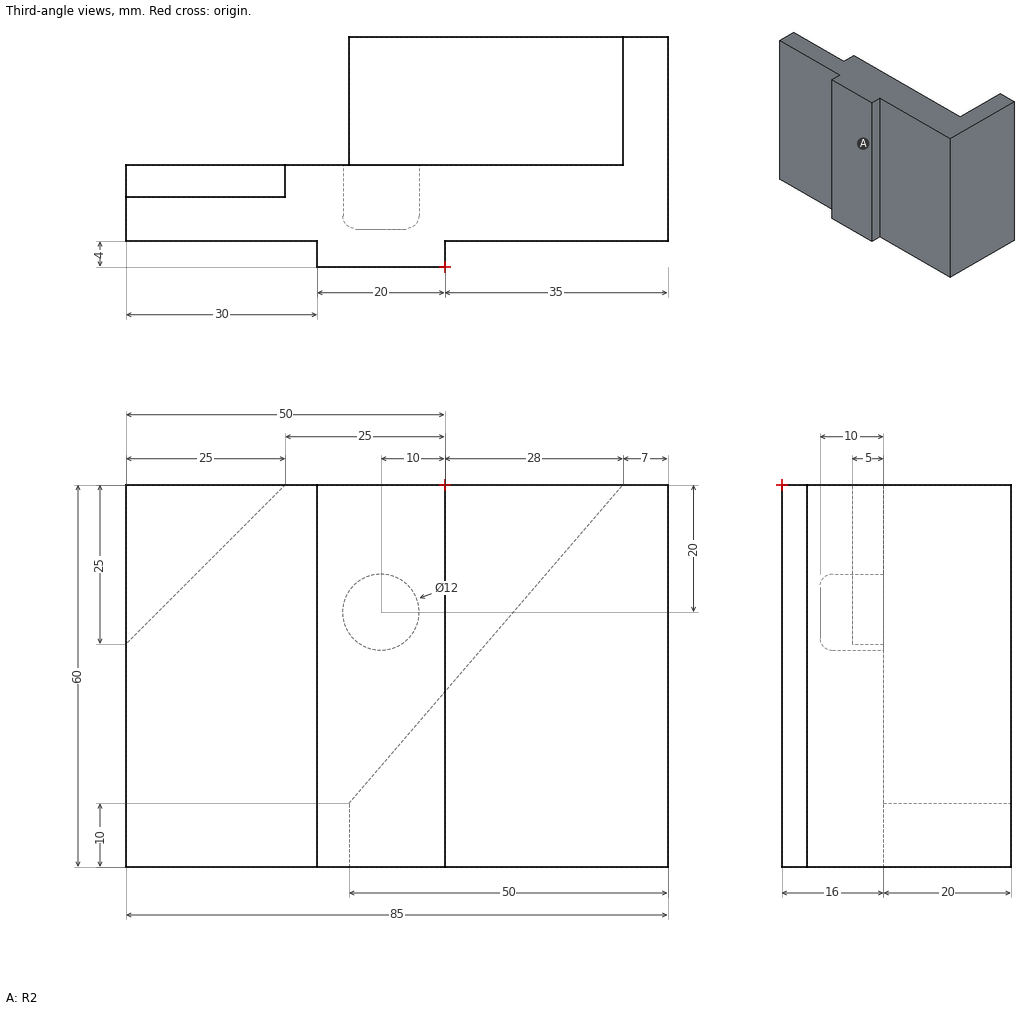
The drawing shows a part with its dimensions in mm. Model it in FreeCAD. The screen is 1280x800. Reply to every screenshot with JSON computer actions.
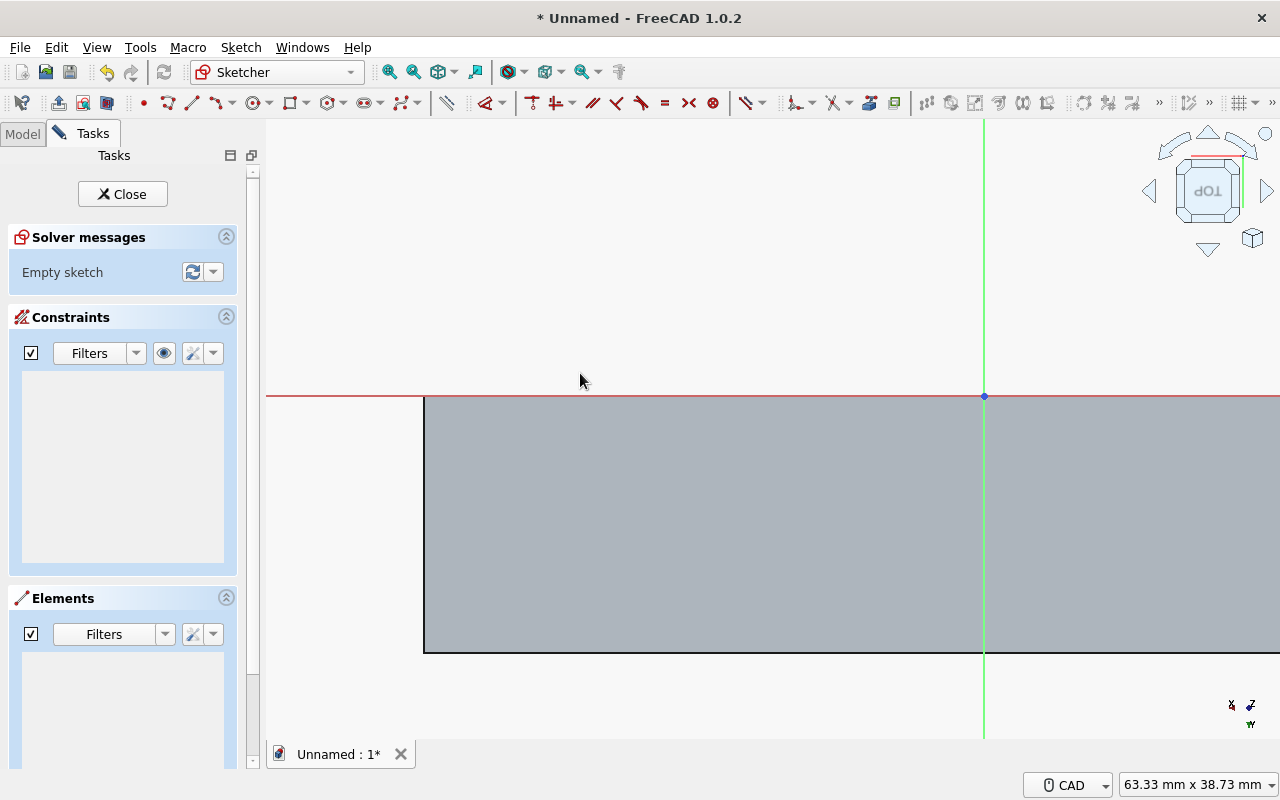
{"action": "left_click", "coordinate": [290, 104]}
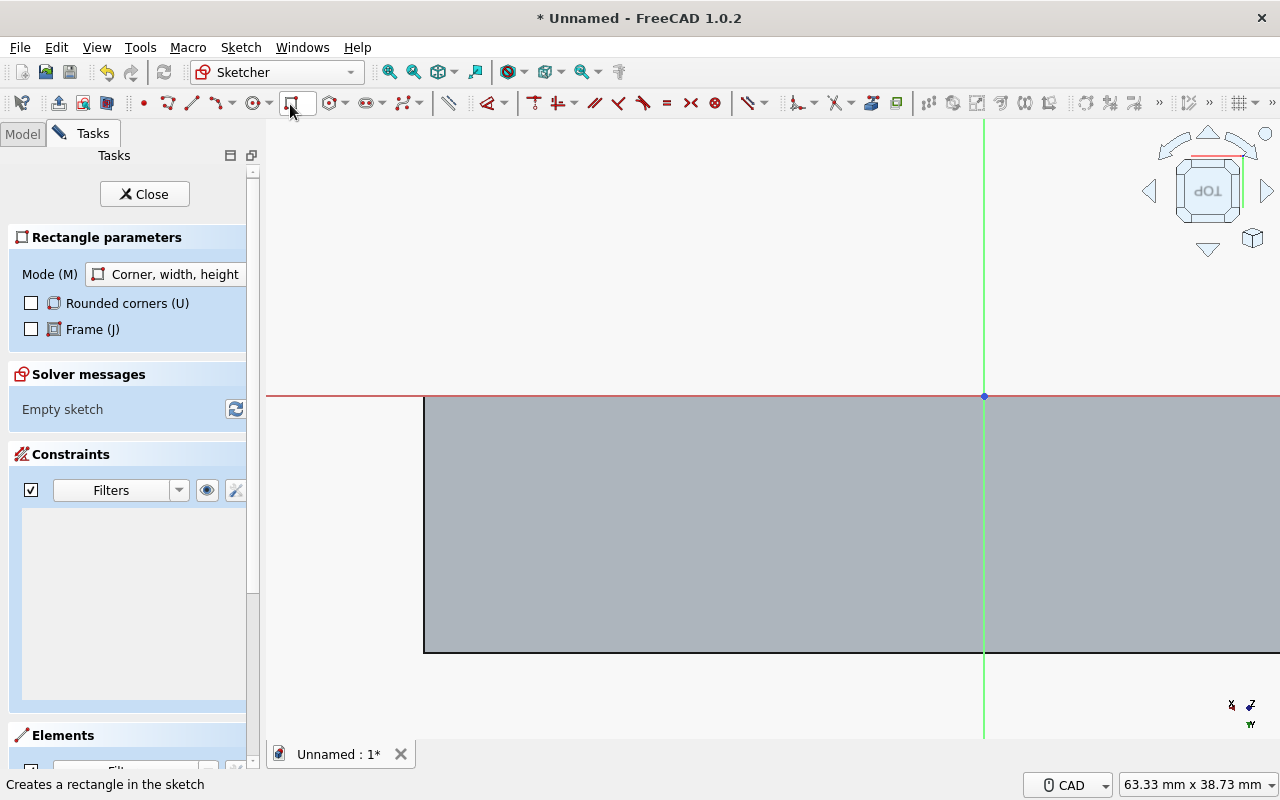
{"action": "left_click", "coordinate": [984, 396]}
{"action": "left_click", "coordinate": [424, 460]}
{"action": "key", "text": "Escape"}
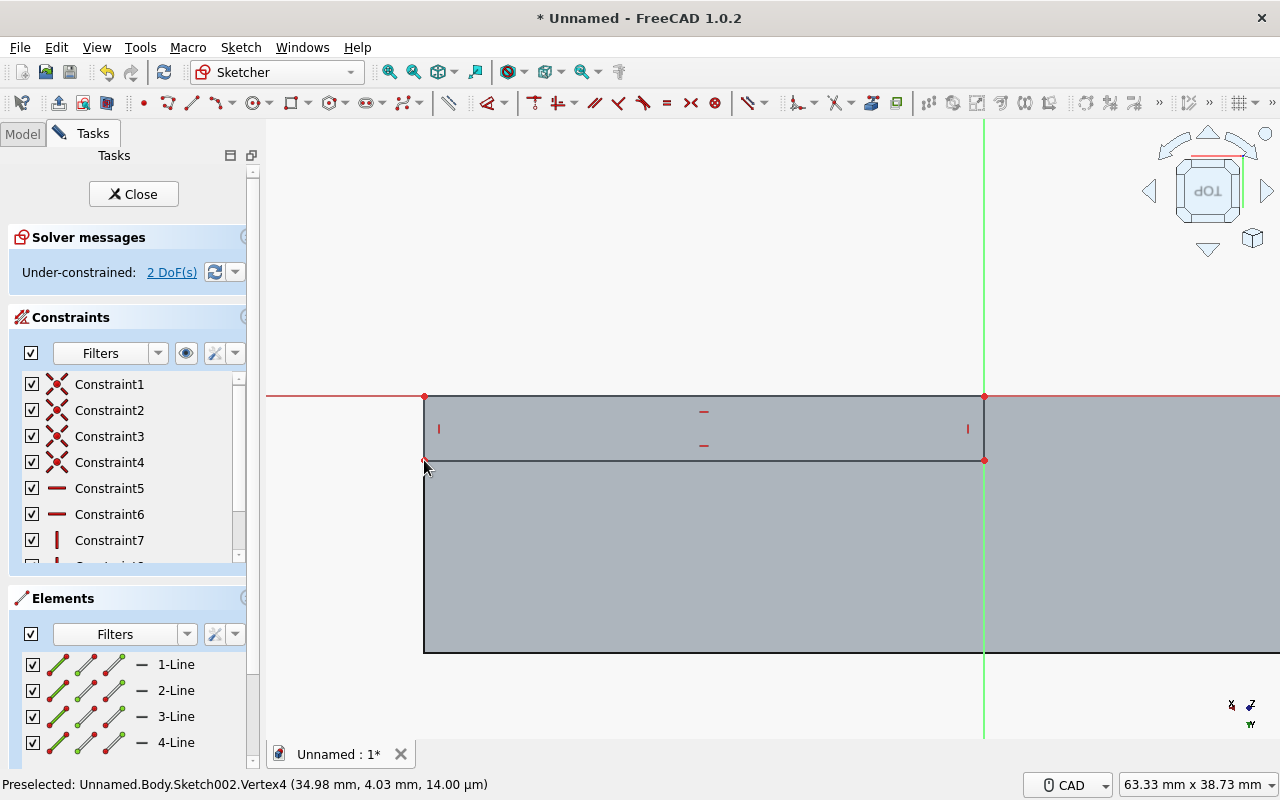
{"action": "left_click", "coordinate": [488, 104]}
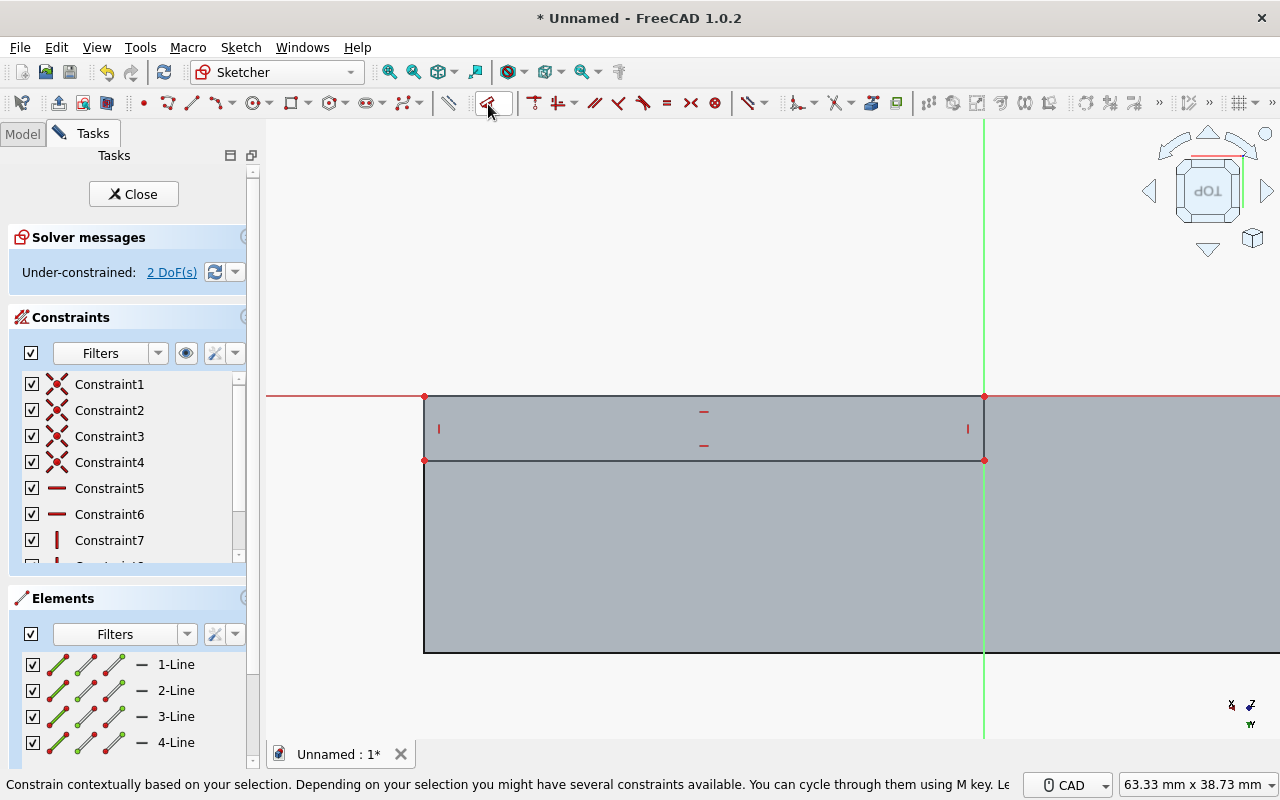
{"action": "left_click", "coordinate": [424, 416]}
{"action": "left_click", "coordinate": [390, 429]}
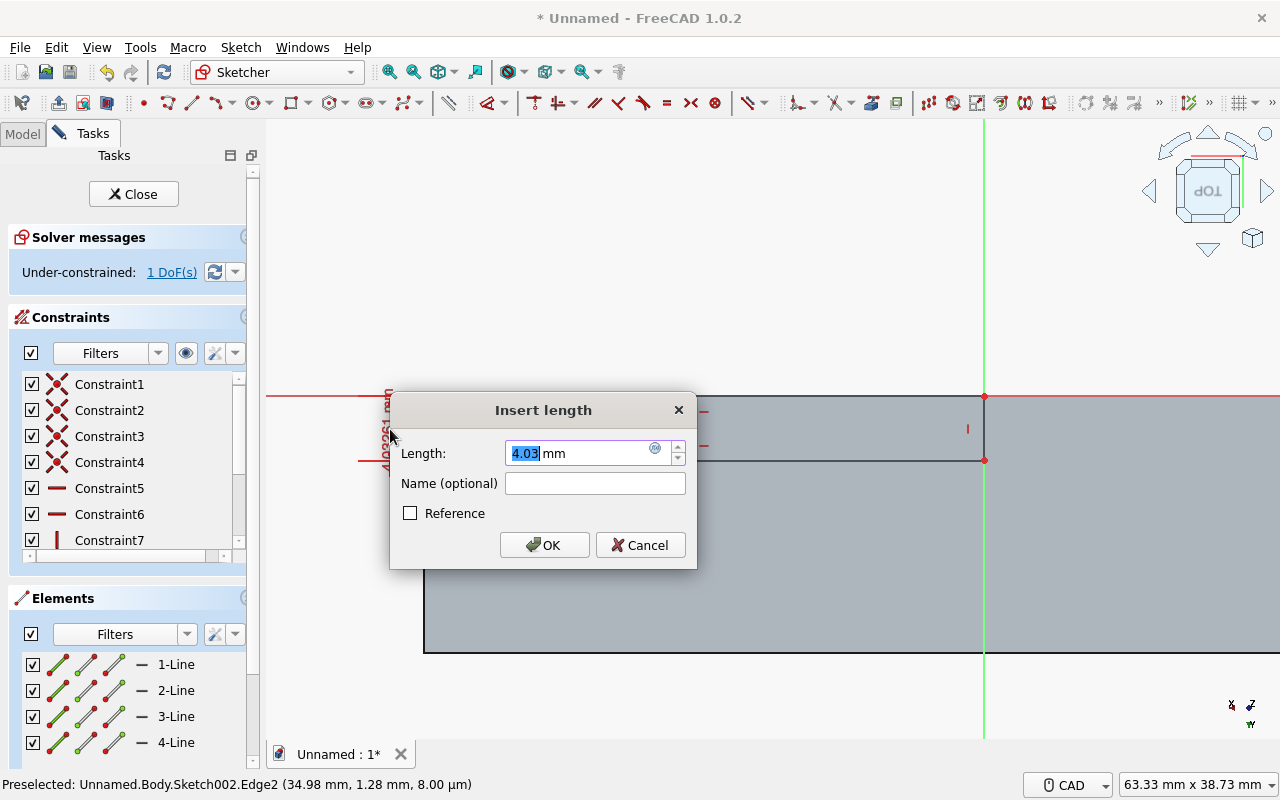
{"action": "type", "text": "4"}
{"action": "key", "text": "Return"}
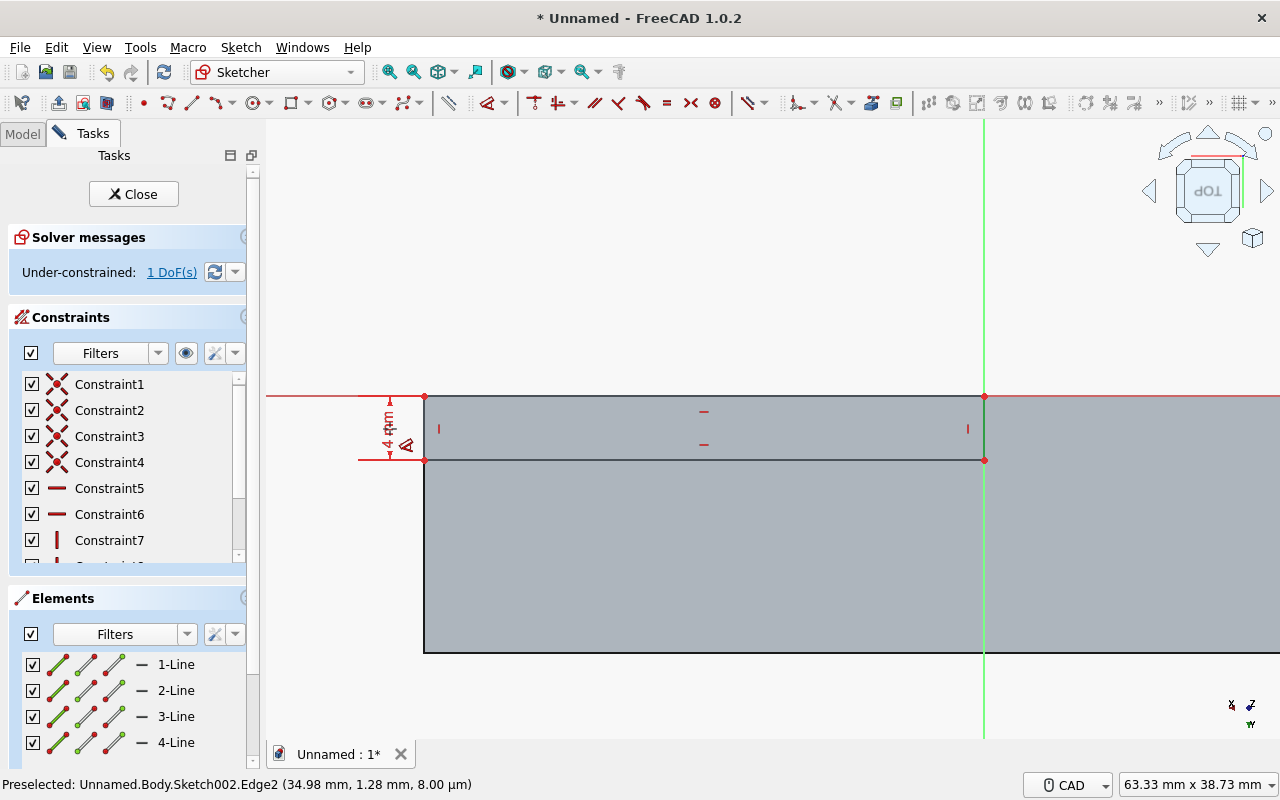
{"action": "left_click", "coordinate": [816, 396]}
{"action": "left_click", "coordinate": [704, 362]}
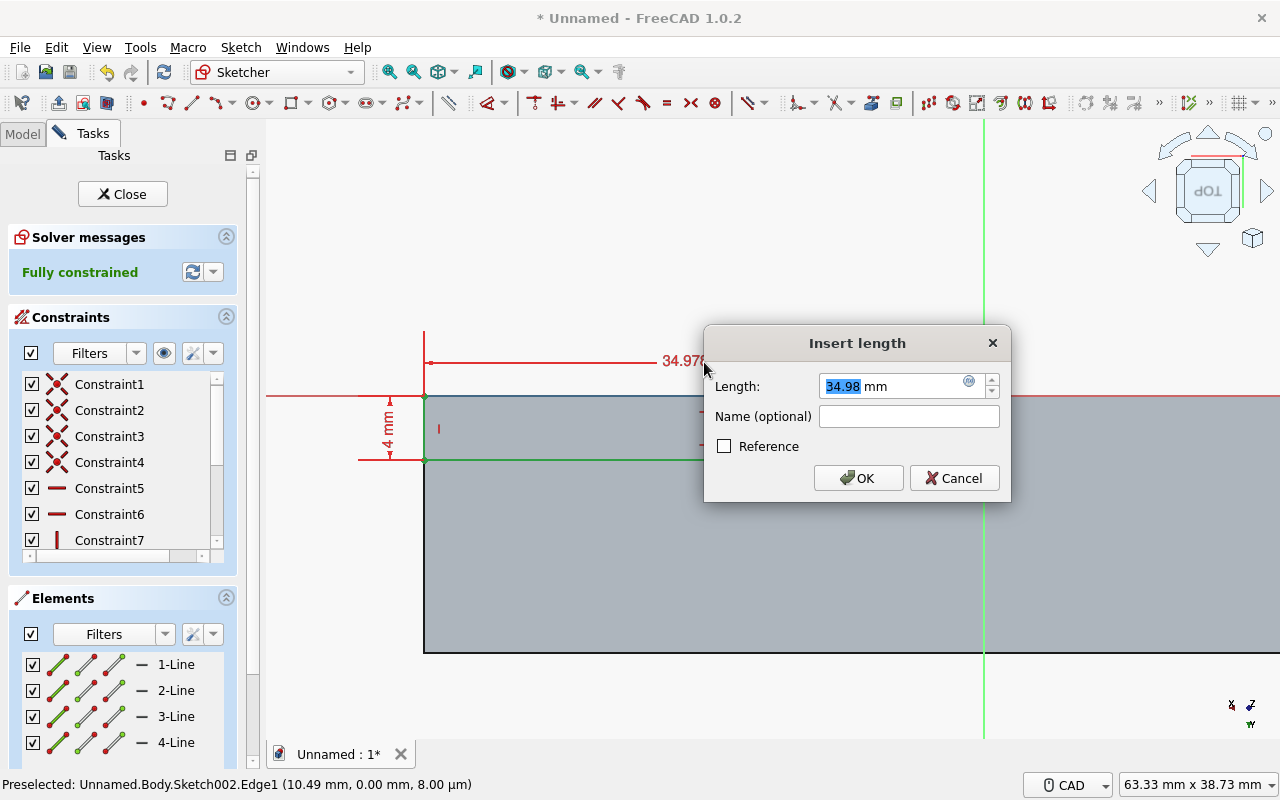
{"action": "type", "text": "35"}
{"action": "key", "text": "Return"}
{"action": "key", "text": "Escape"}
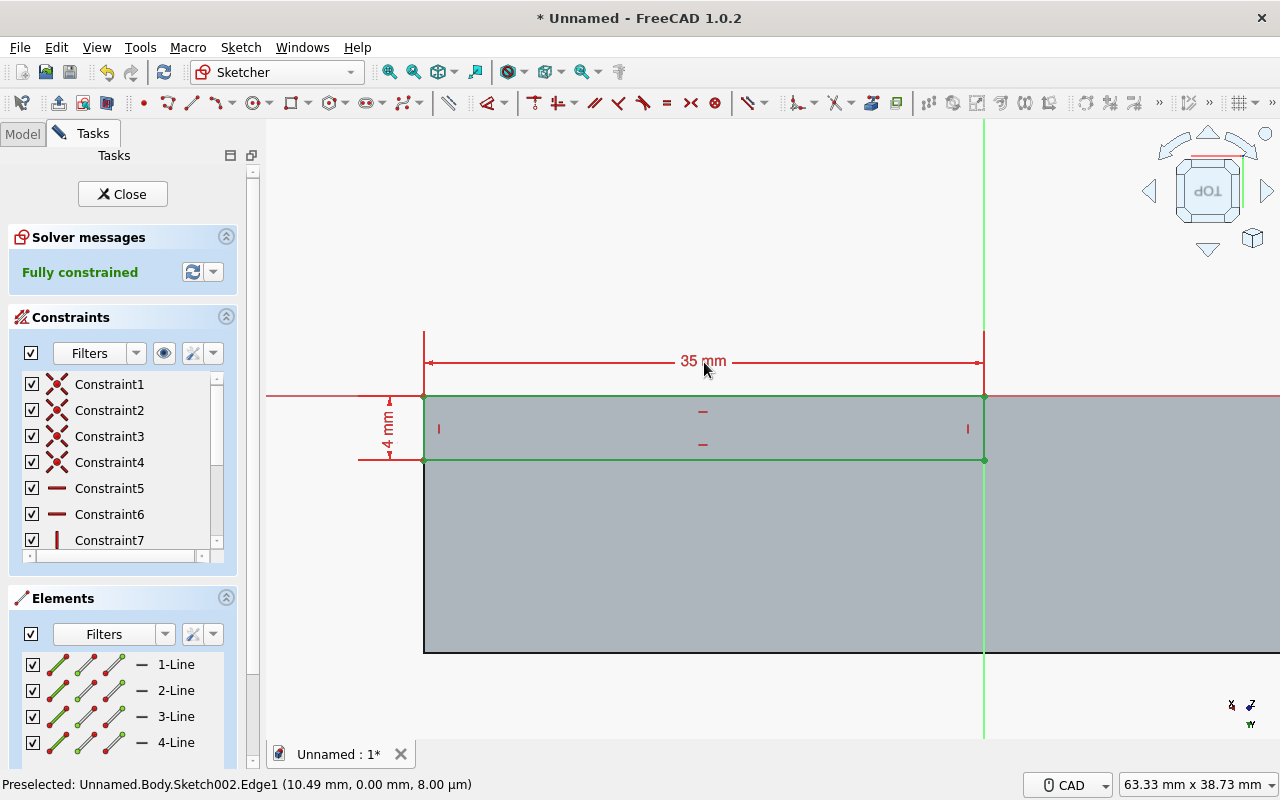
{"action": "left_click", "coordinate": [123, 194]}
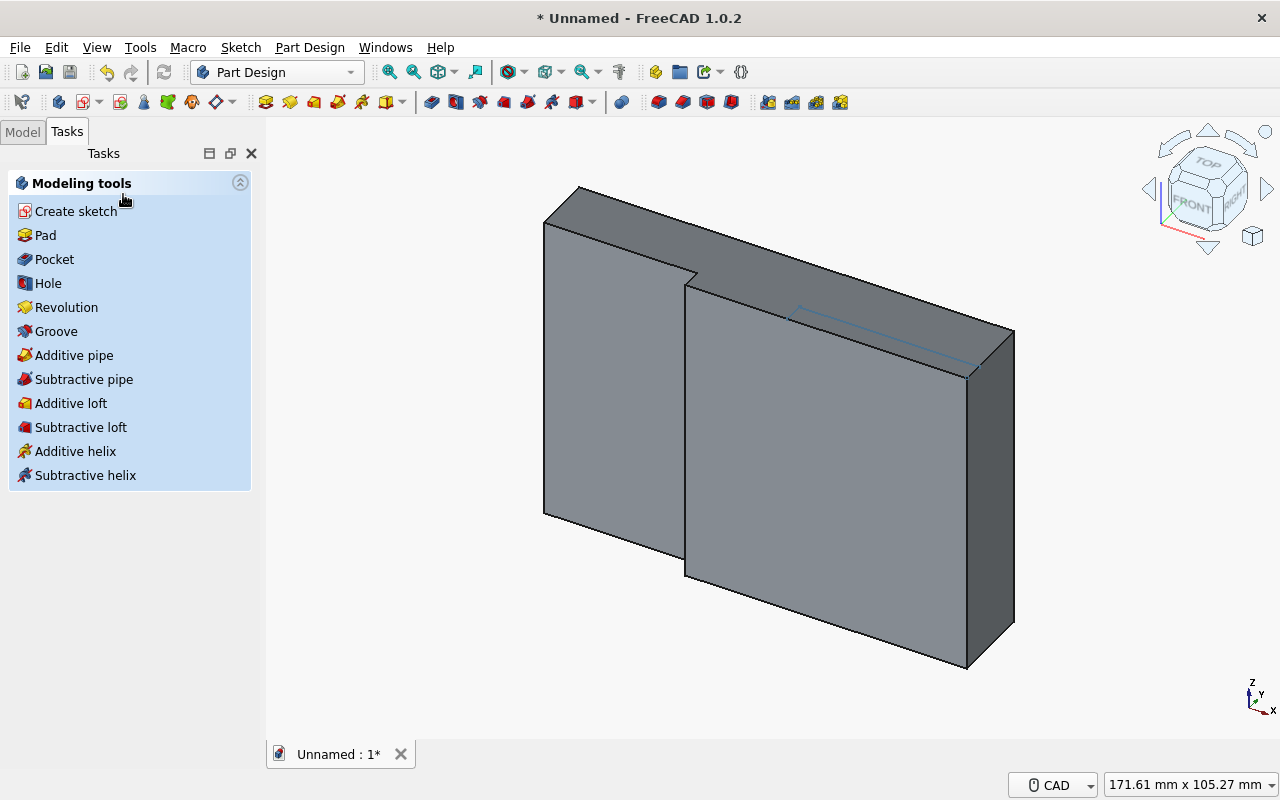
{"action": "left_click", "coordinate": [432, 102]}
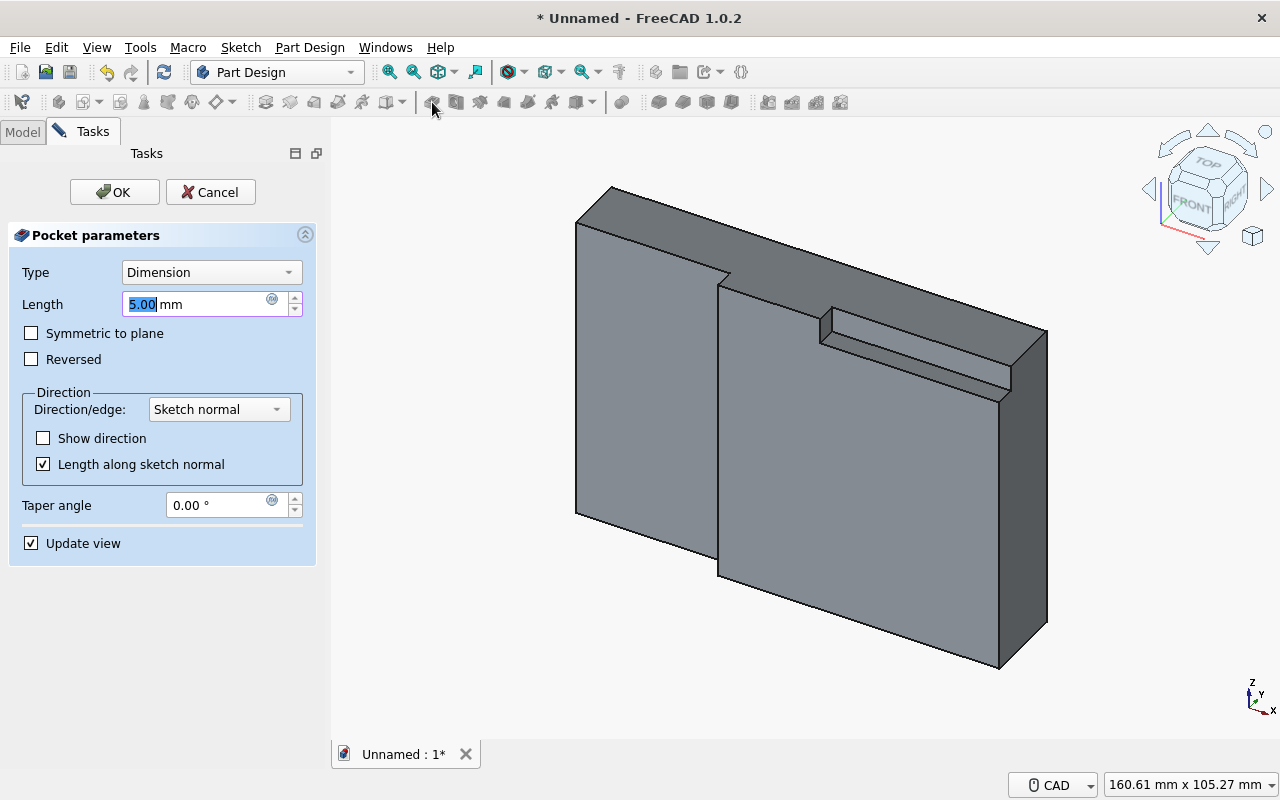
{"action": "left_click", "coordinate": [212, 272]}